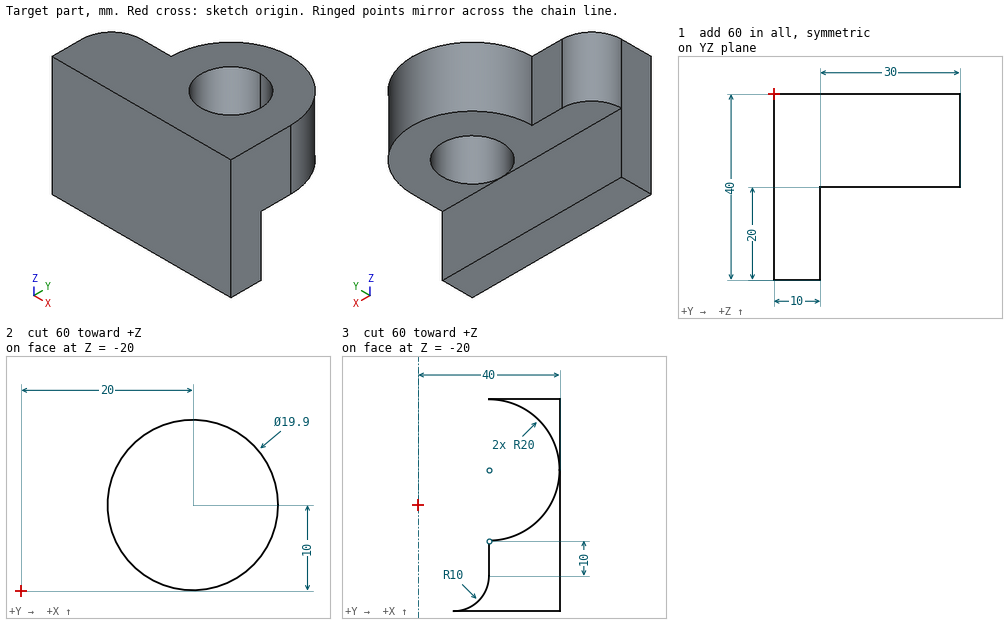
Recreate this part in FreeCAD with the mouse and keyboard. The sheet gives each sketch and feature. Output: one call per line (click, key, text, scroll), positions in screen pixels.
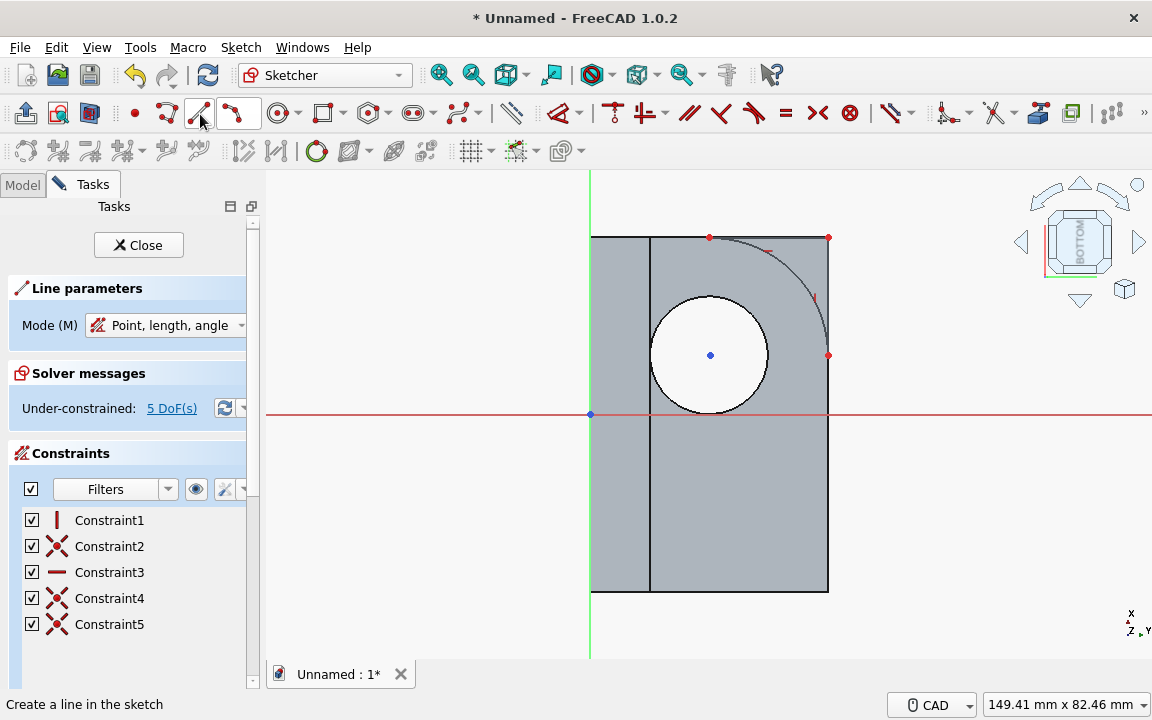
click(709, 474)
click(709, 533)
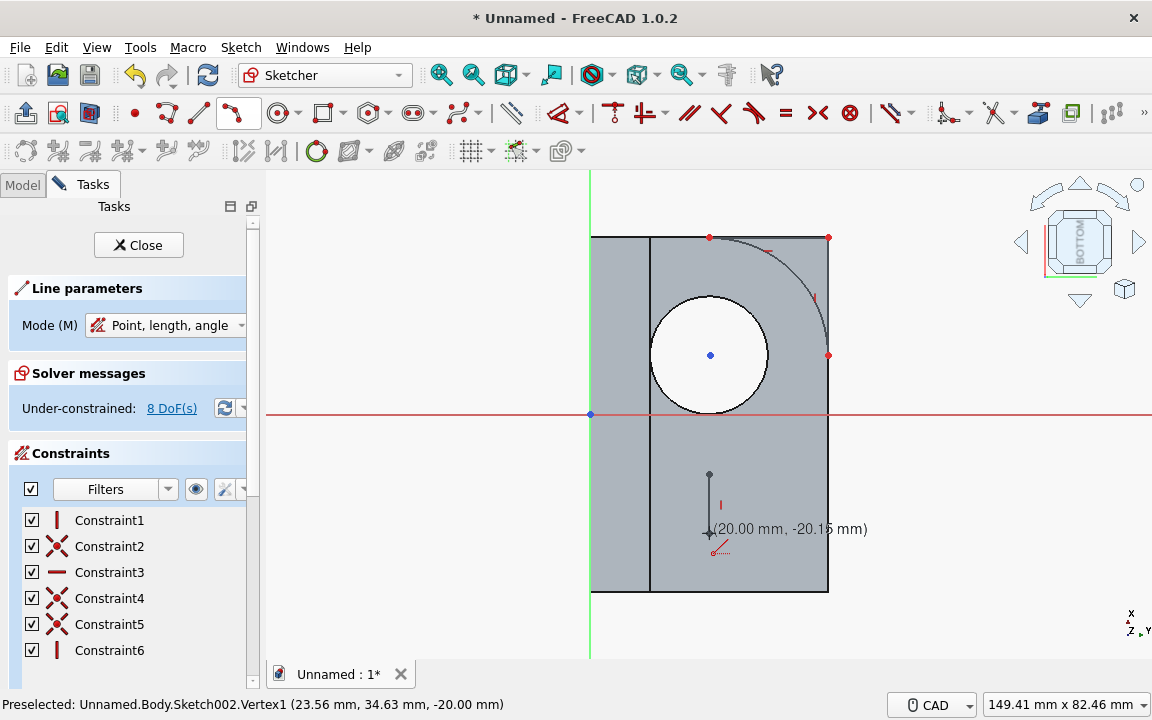
click(168, 114)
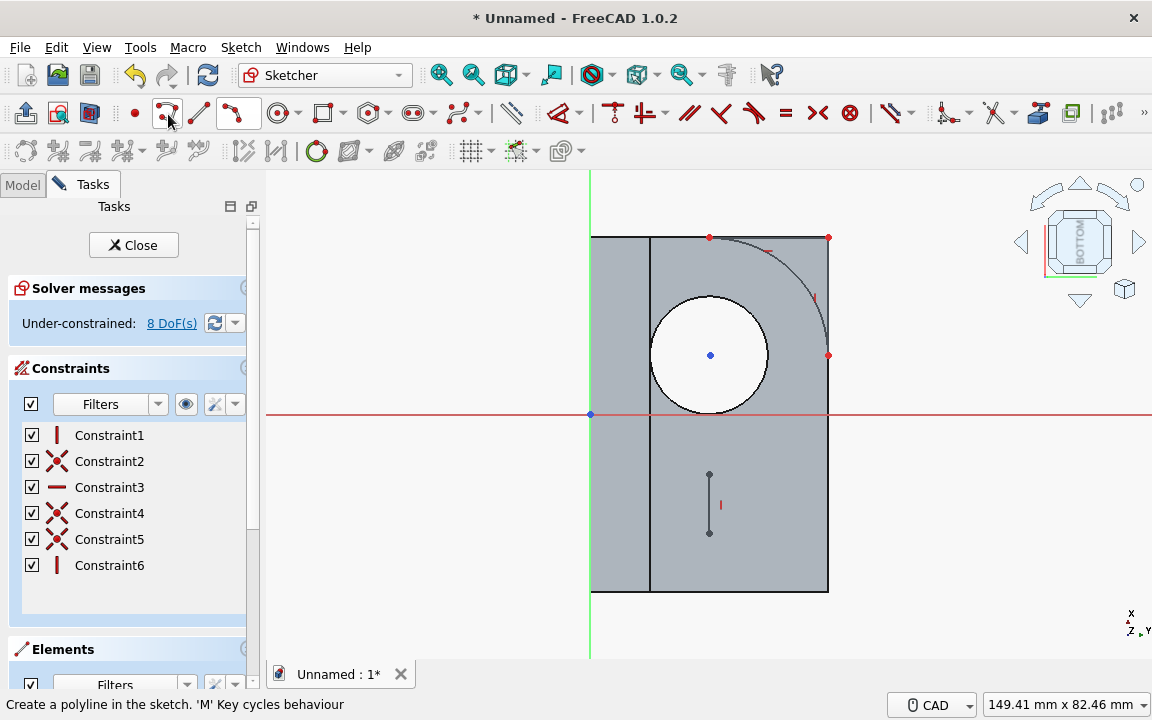
click(650, 592)
click(828, 592)
click(828, 356)
right_click(828, 592)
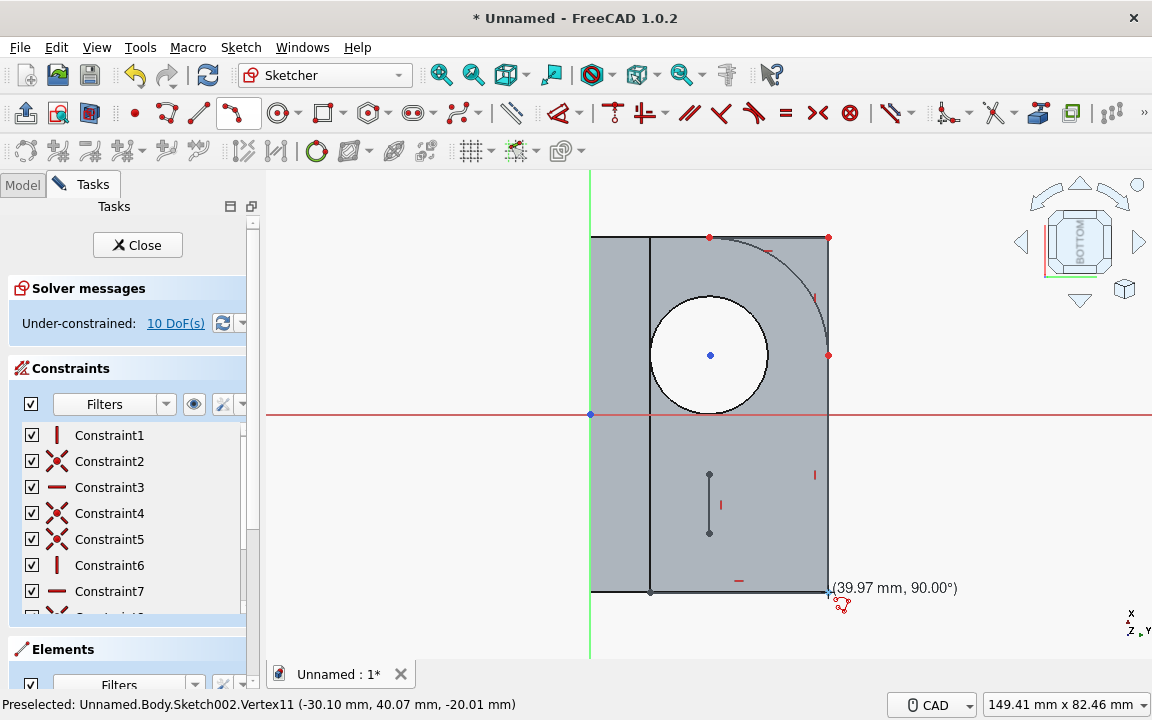
click(232, 114)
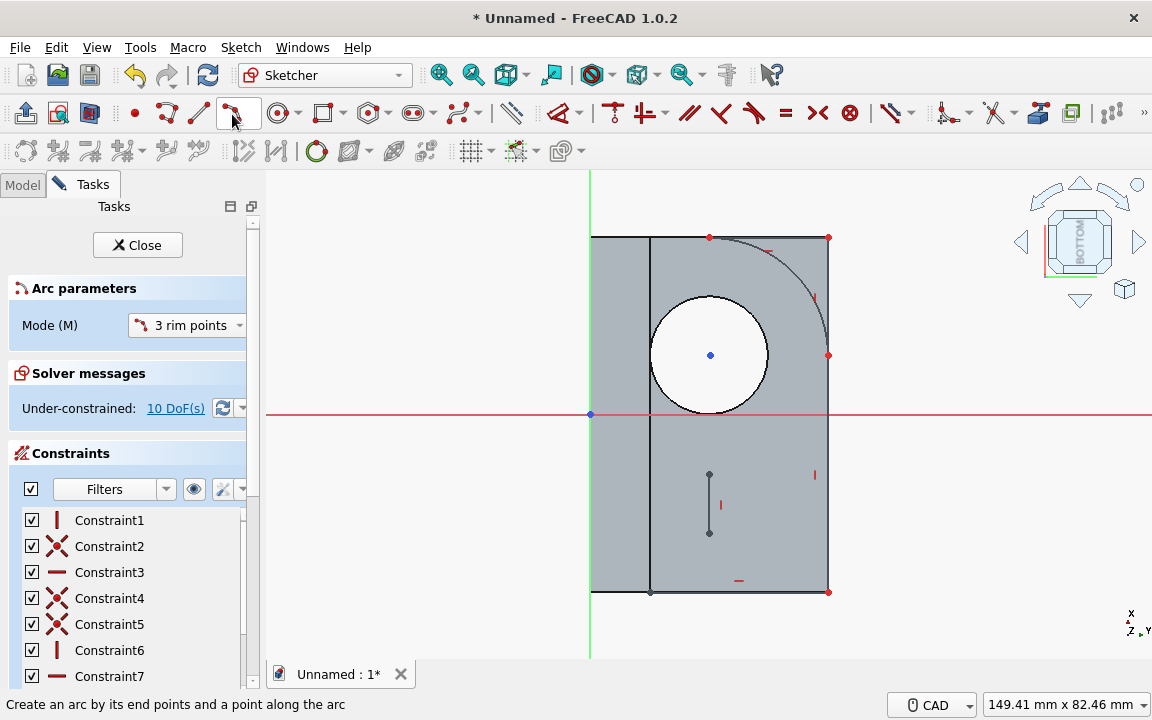
click(709, 534)
click(650, 593)
click(692, 575)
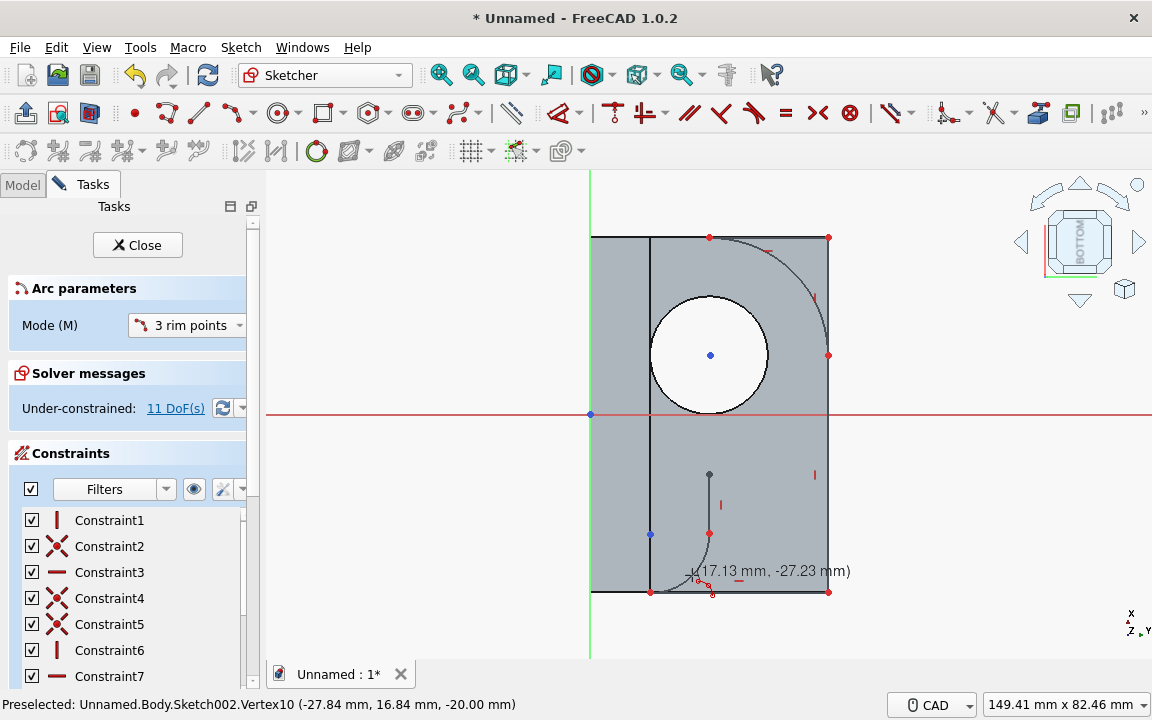
click(828, 356)
click(709, 475)
click(793, 439)
key(Escape)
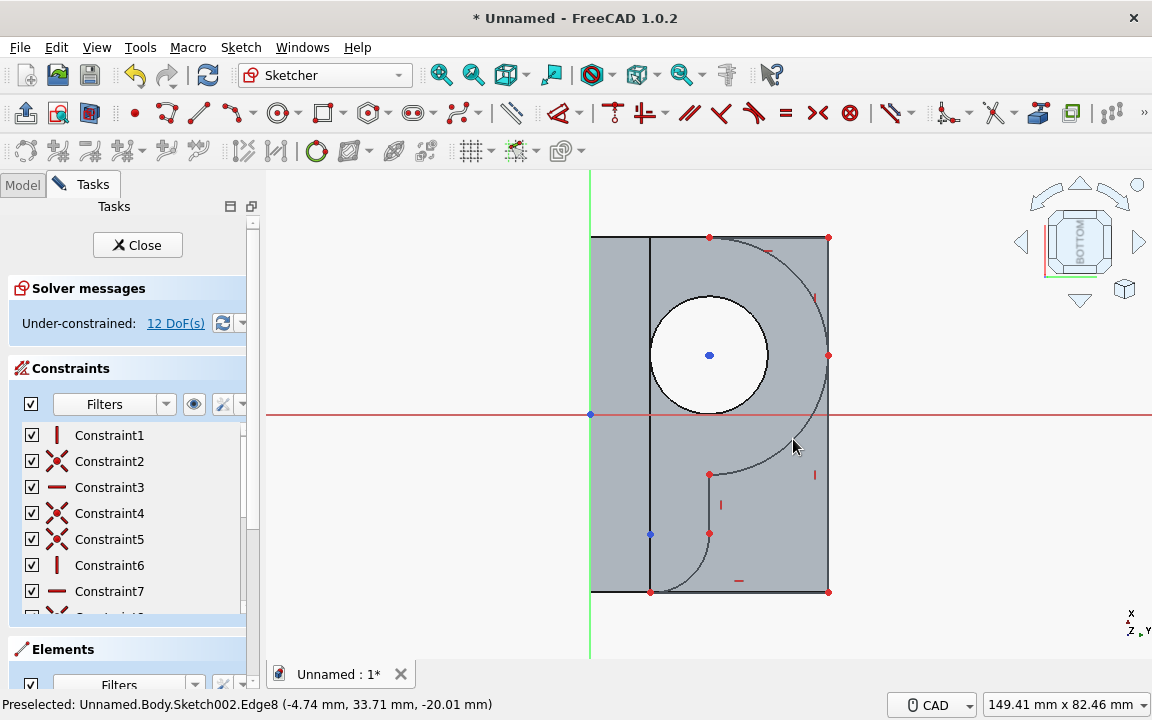
click(828, 273)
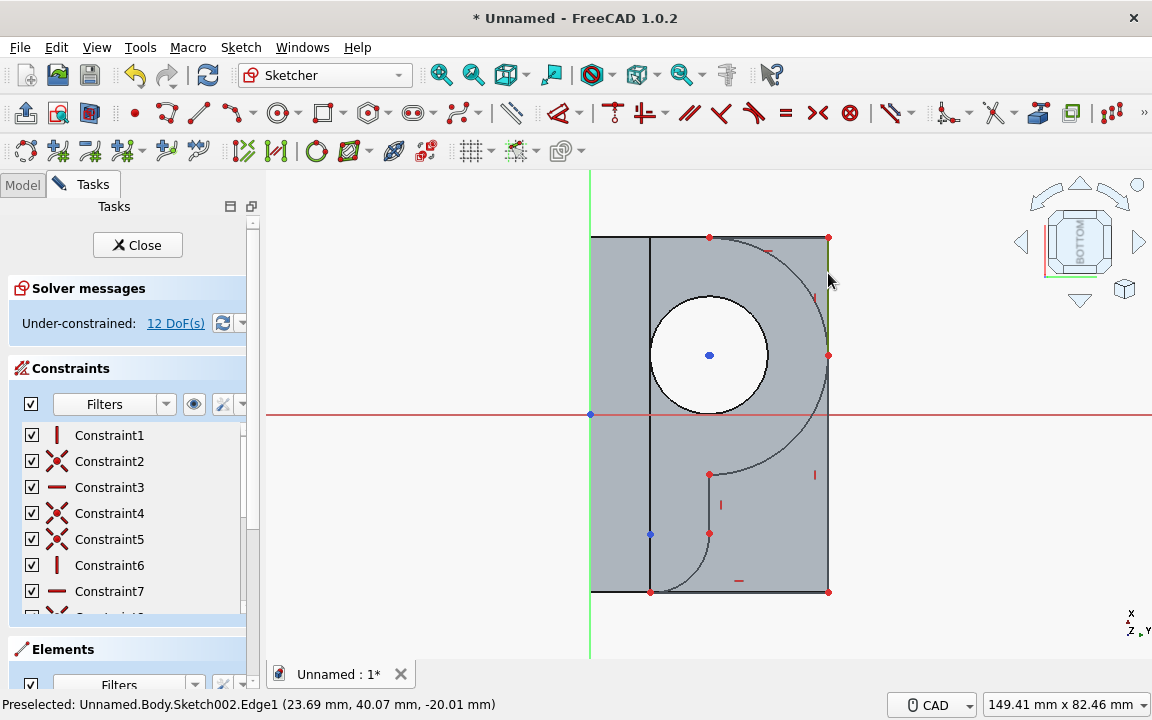
click(793, 272)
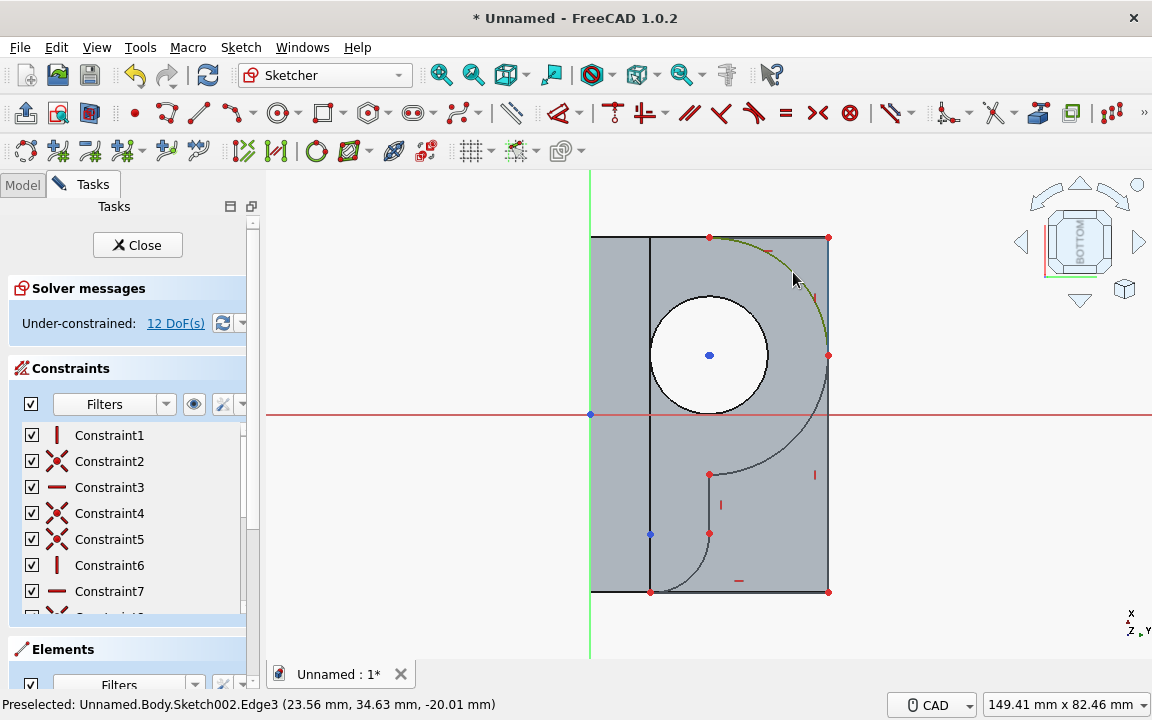
click(754, 114)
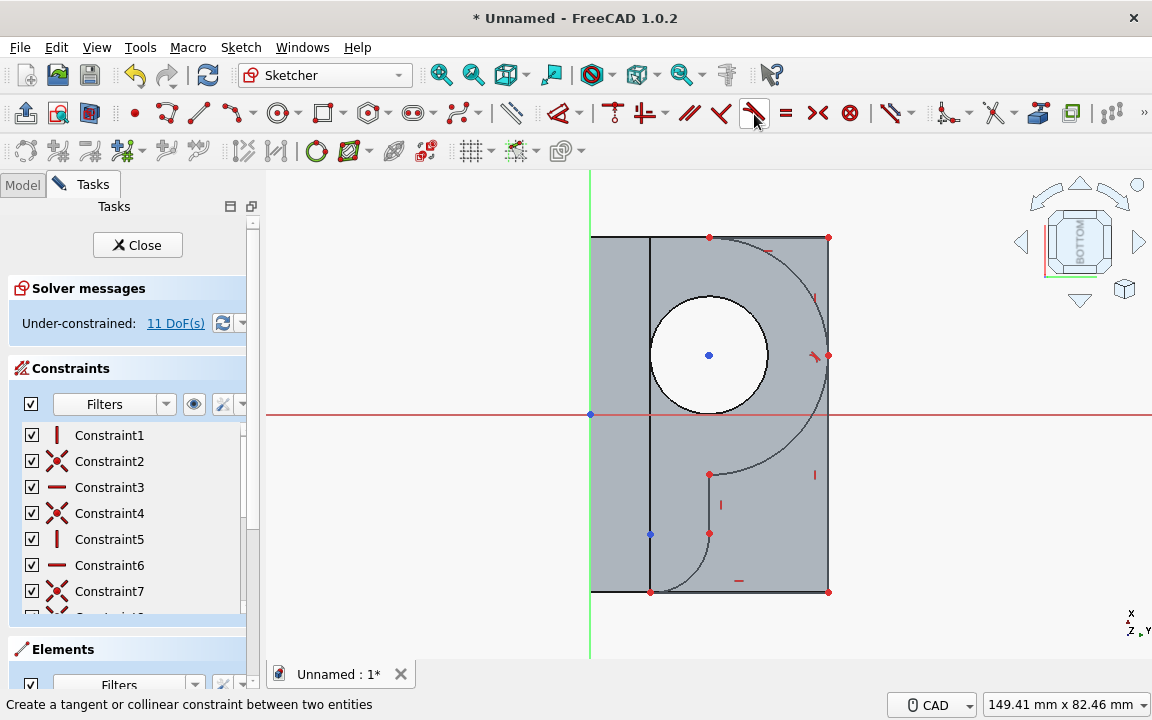
click(828, 273)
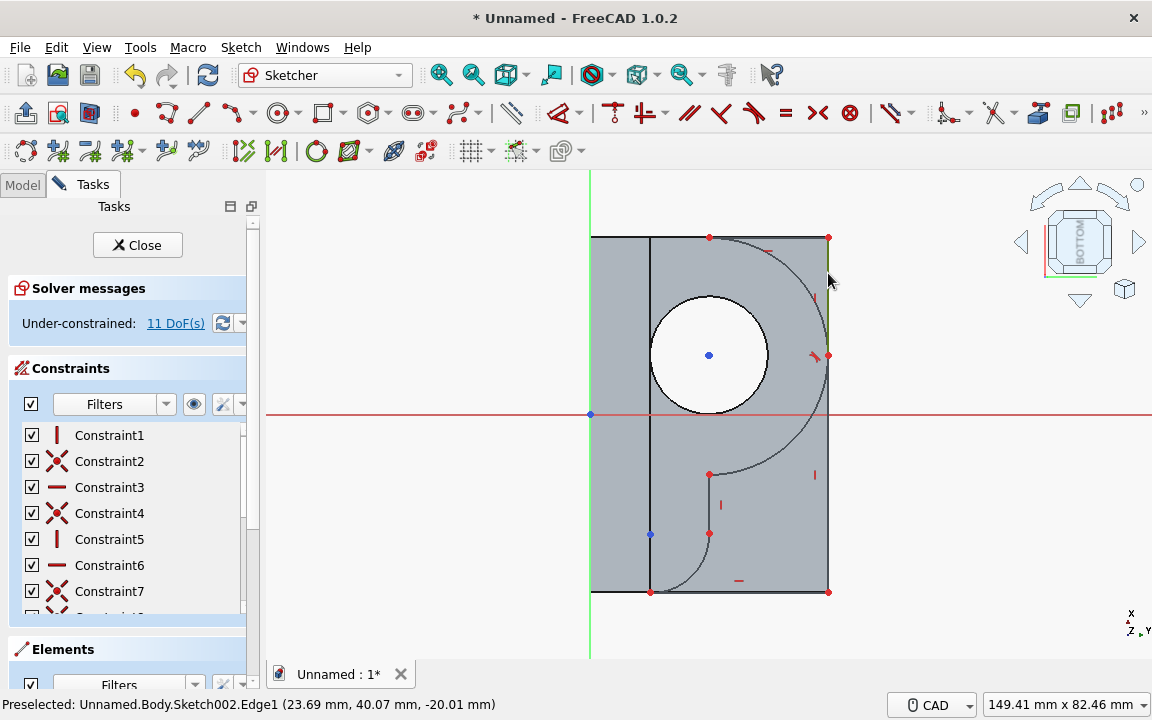
click(763, 462)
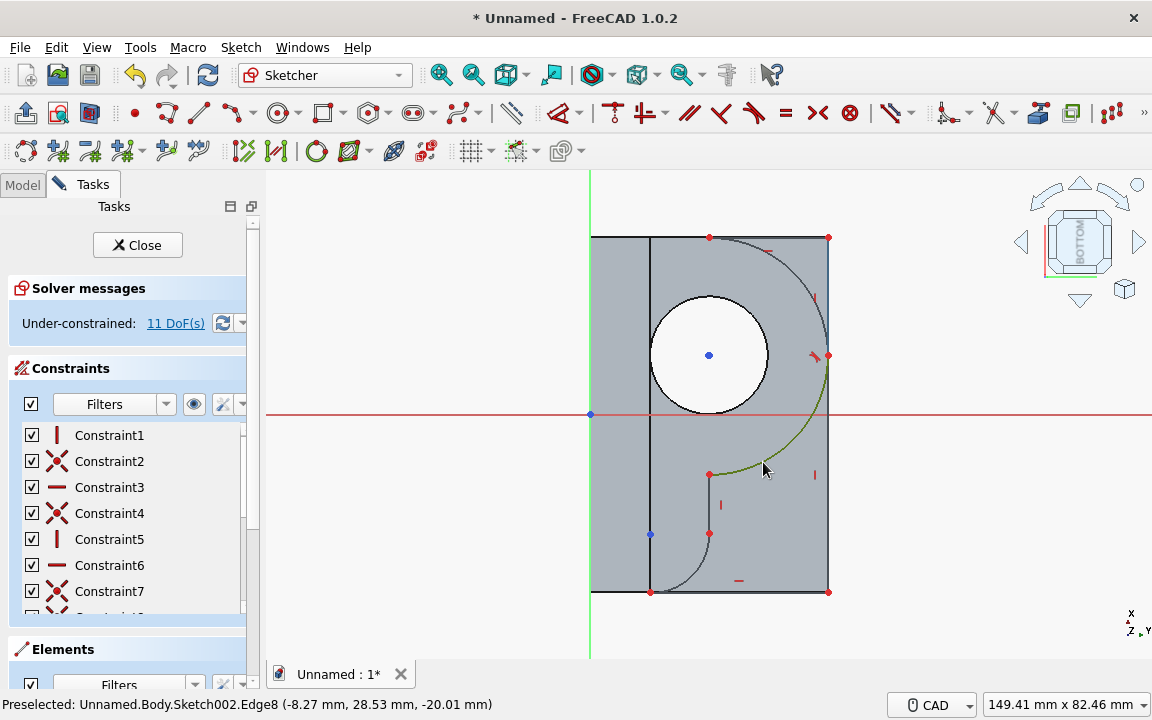
click(754, 114)